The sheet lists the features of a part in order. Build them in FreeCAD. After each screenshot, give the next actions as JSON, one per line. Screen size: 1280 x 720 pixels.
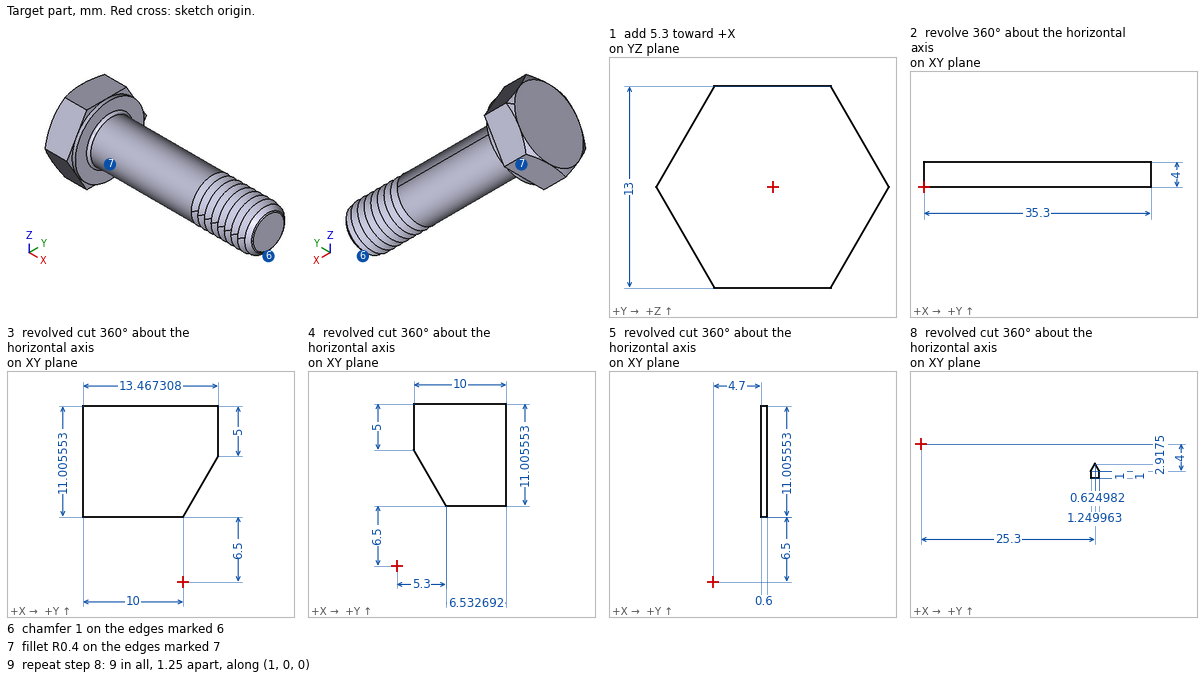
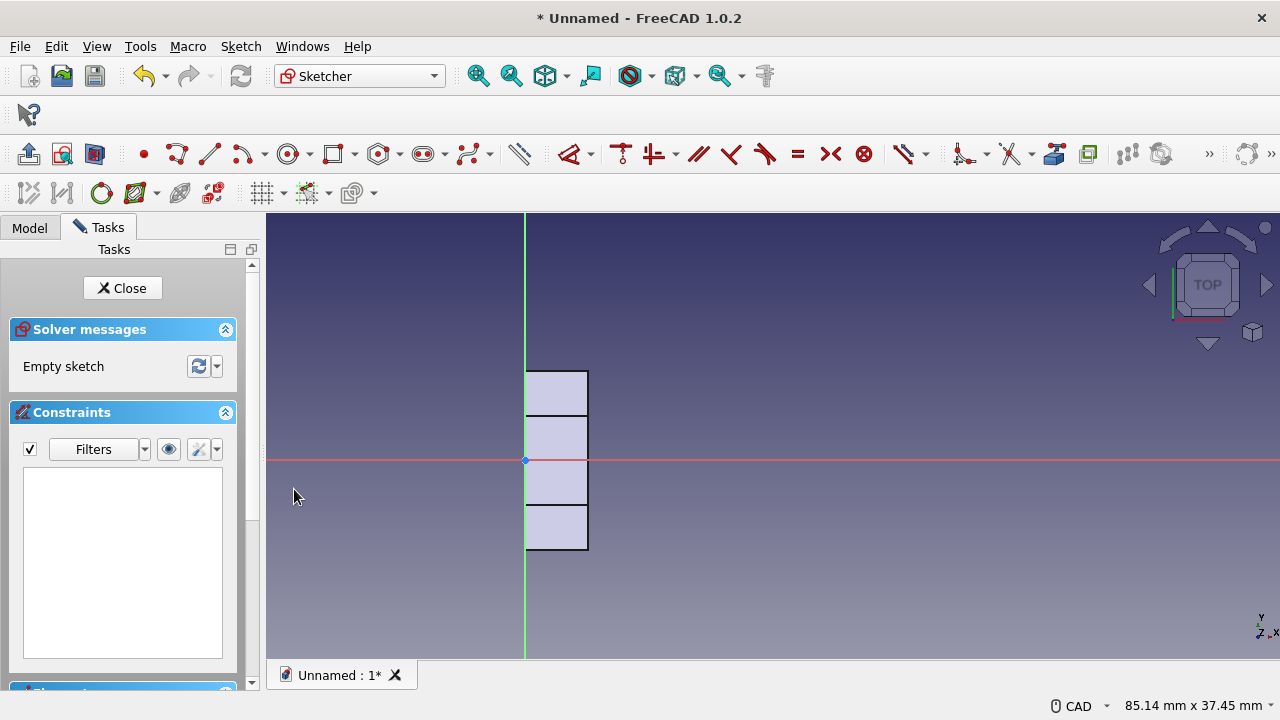
{"action": "scroll", "coordinate": [799, 437], "scroll_direction": "up", "scroll_amount": 2}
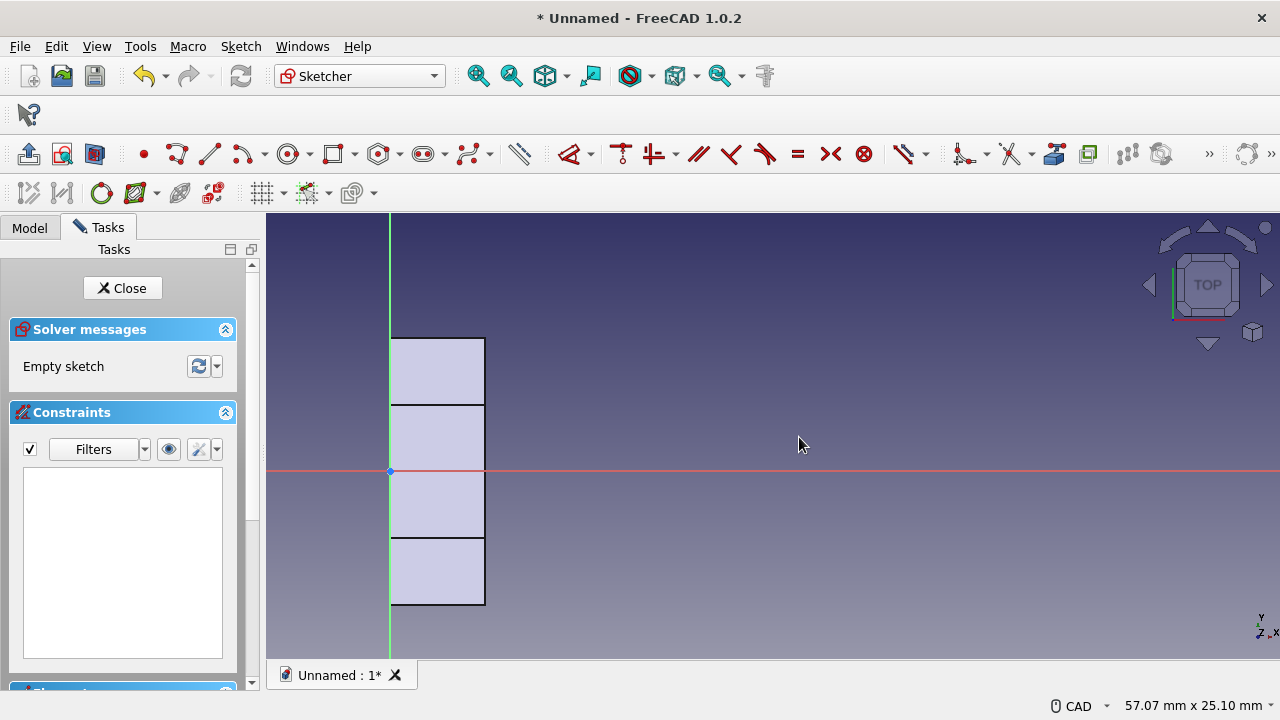
{"action": "left_click", "coordinate": [332, 154]}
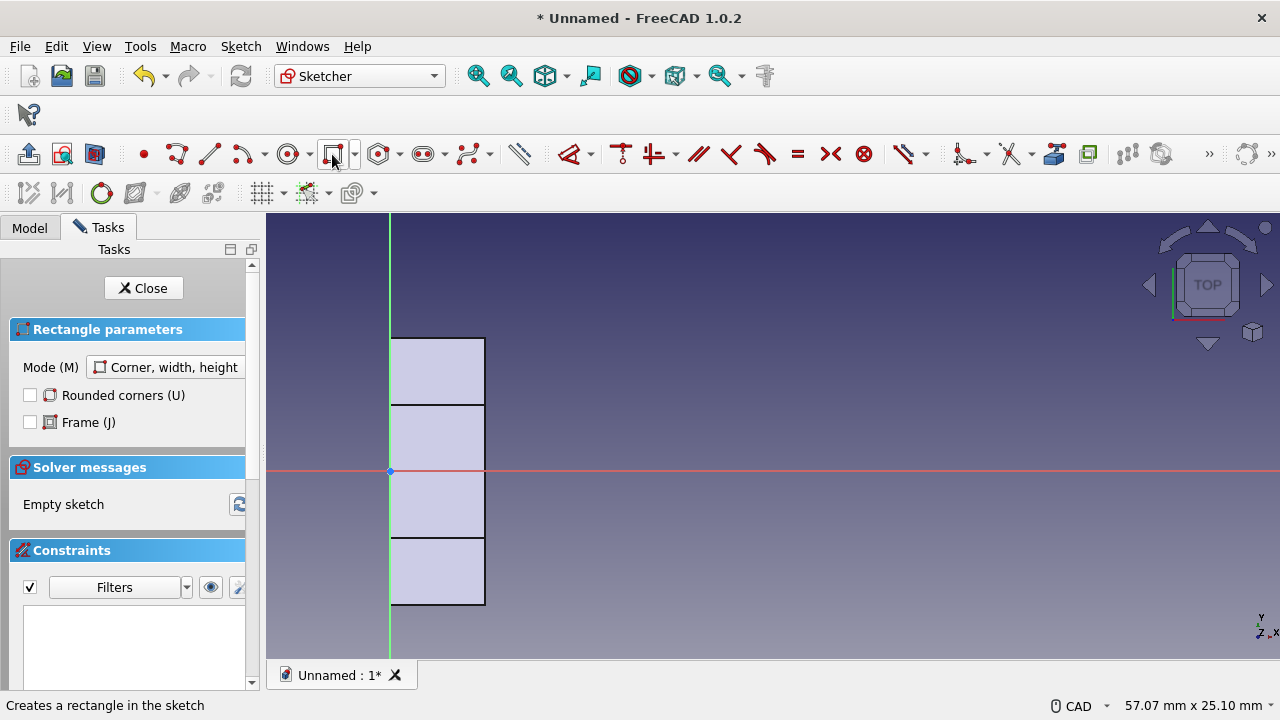
{"action": "left_click", "coordinate": [390, 471]}
{"action": "mouse_move", "coordinate": [1018, 400]}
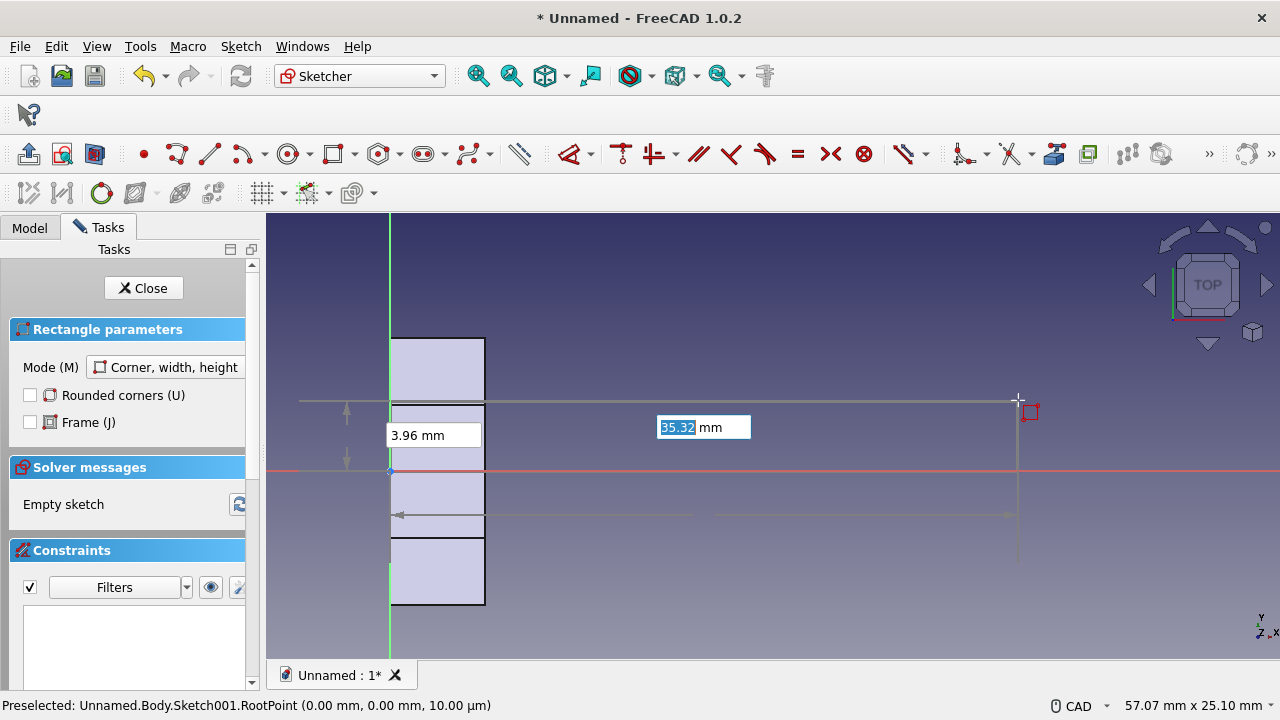
{"action": "type", "text": "35.3"}
{"action": "key", "text": "Tab"}
{"action": "type", "text": "4"}
{"action": "key", "text": "Return"}
{"action": "key", "text": "Escape"}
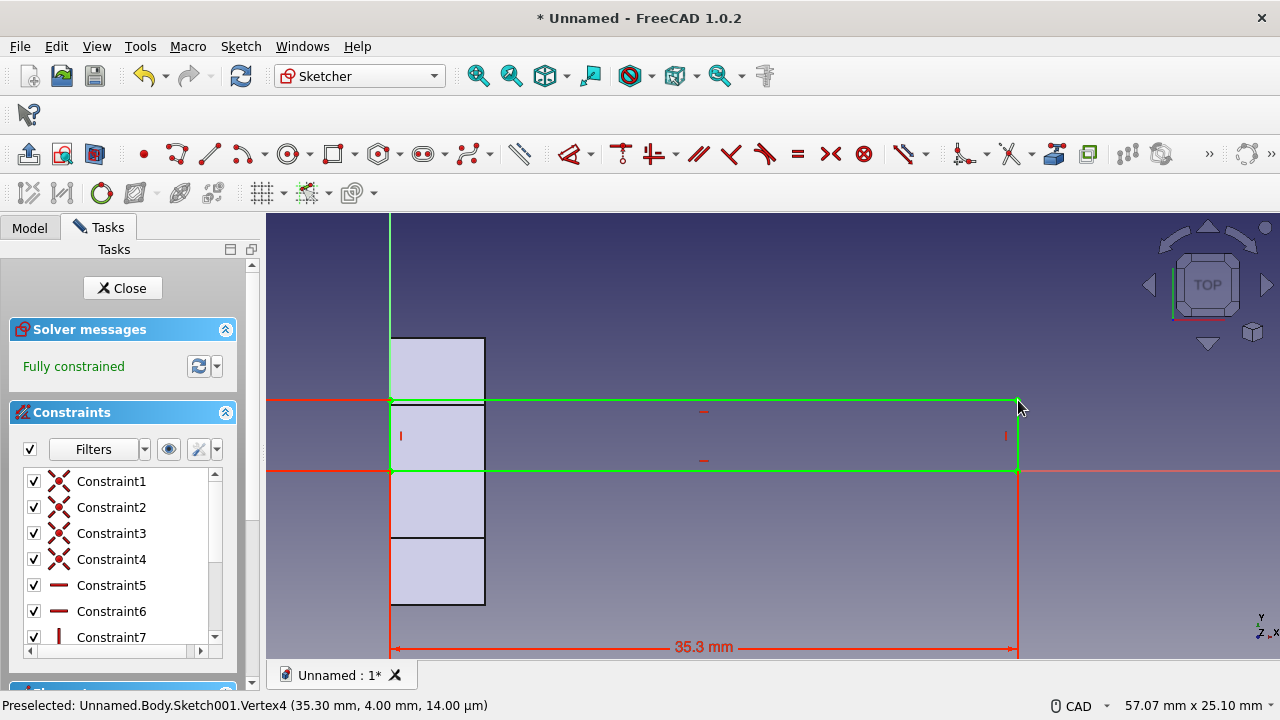
{"action": "left_click", "coordinate": [123, 288]}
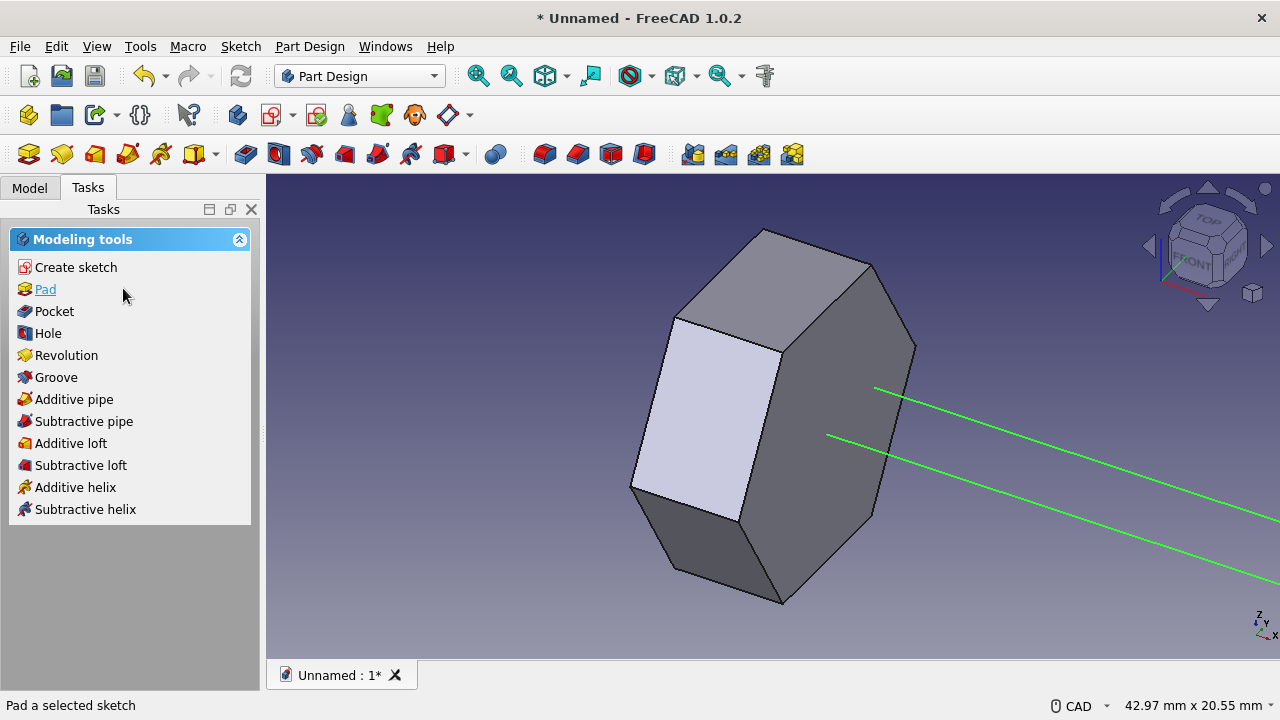
{"action": "left_click", "coordinate": [62, 154]}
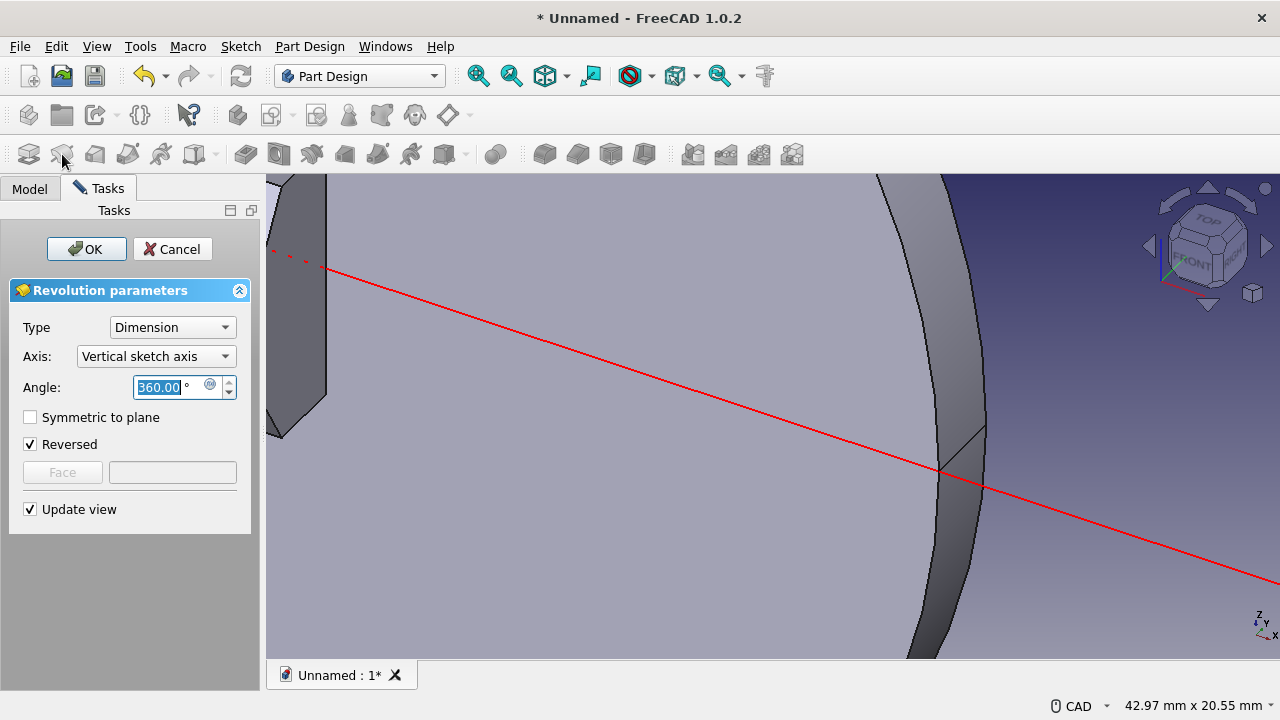
{"action": "left_click", "coordinate": [157, 356]}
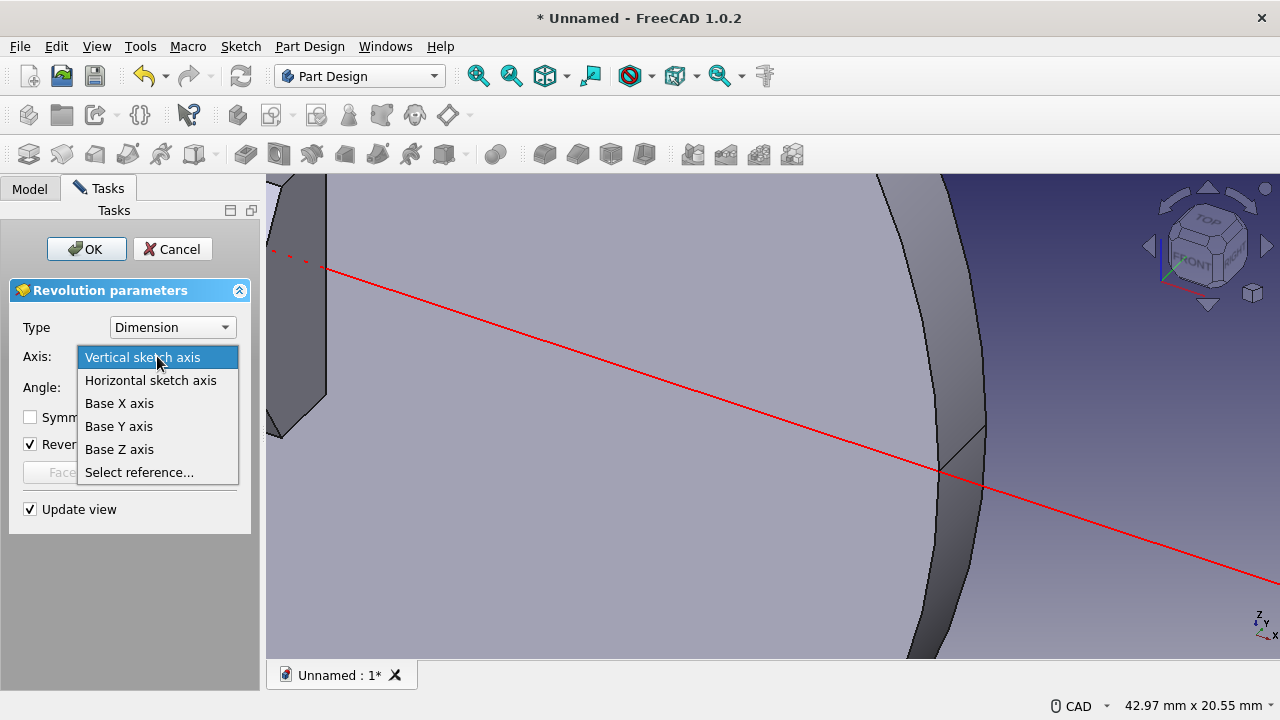
{"action": "left_click", "coordinate": [156, 380]}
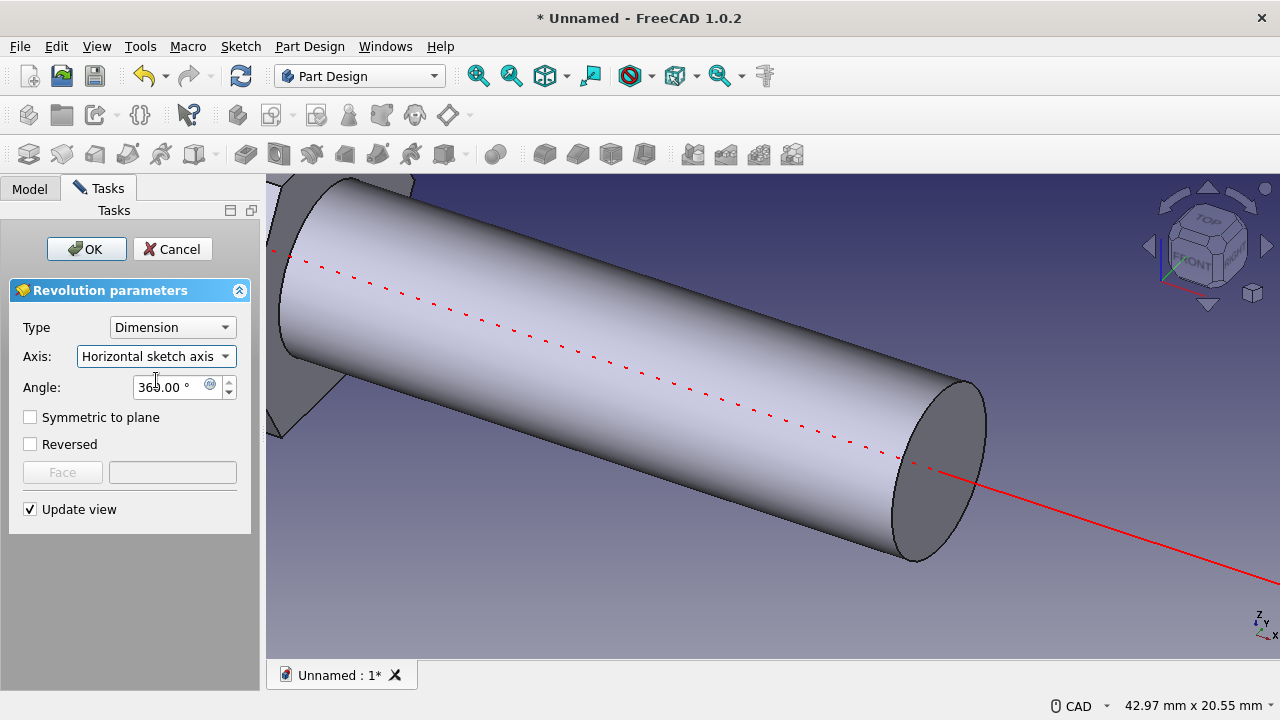
{"action": "left_click", "coordinate": [87, 249]}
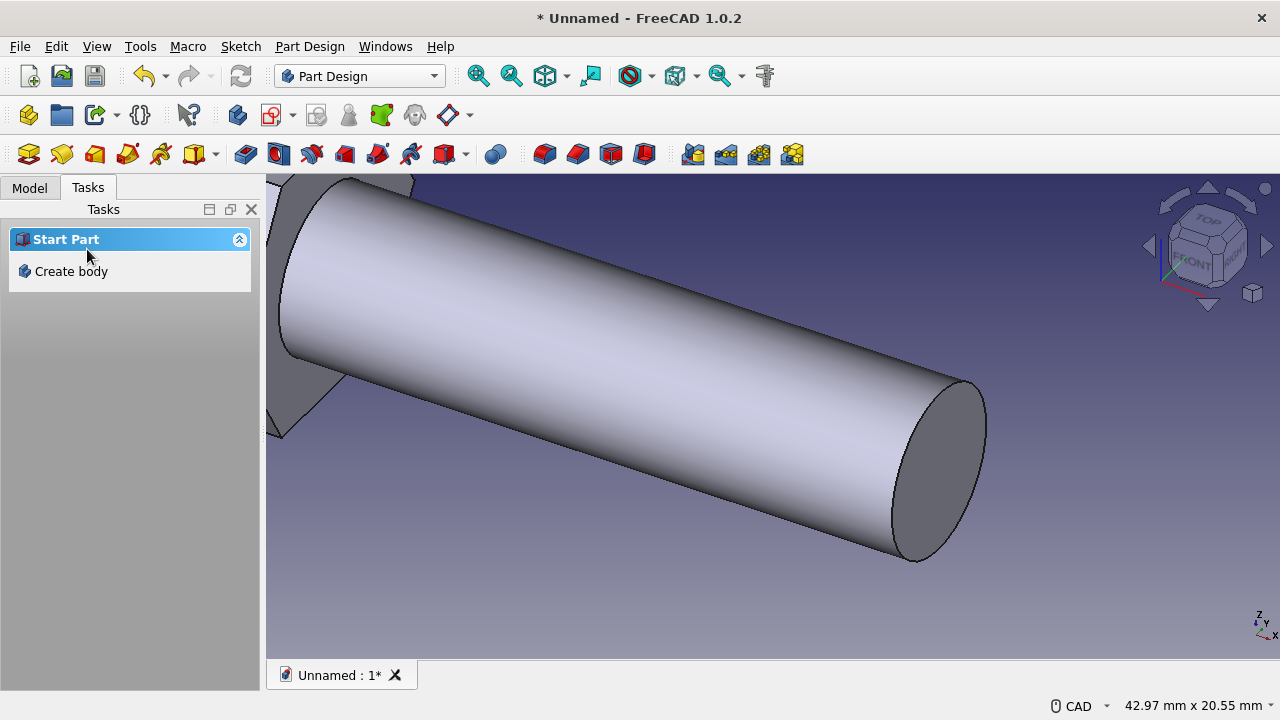
{"action": "key", "text": "v f"}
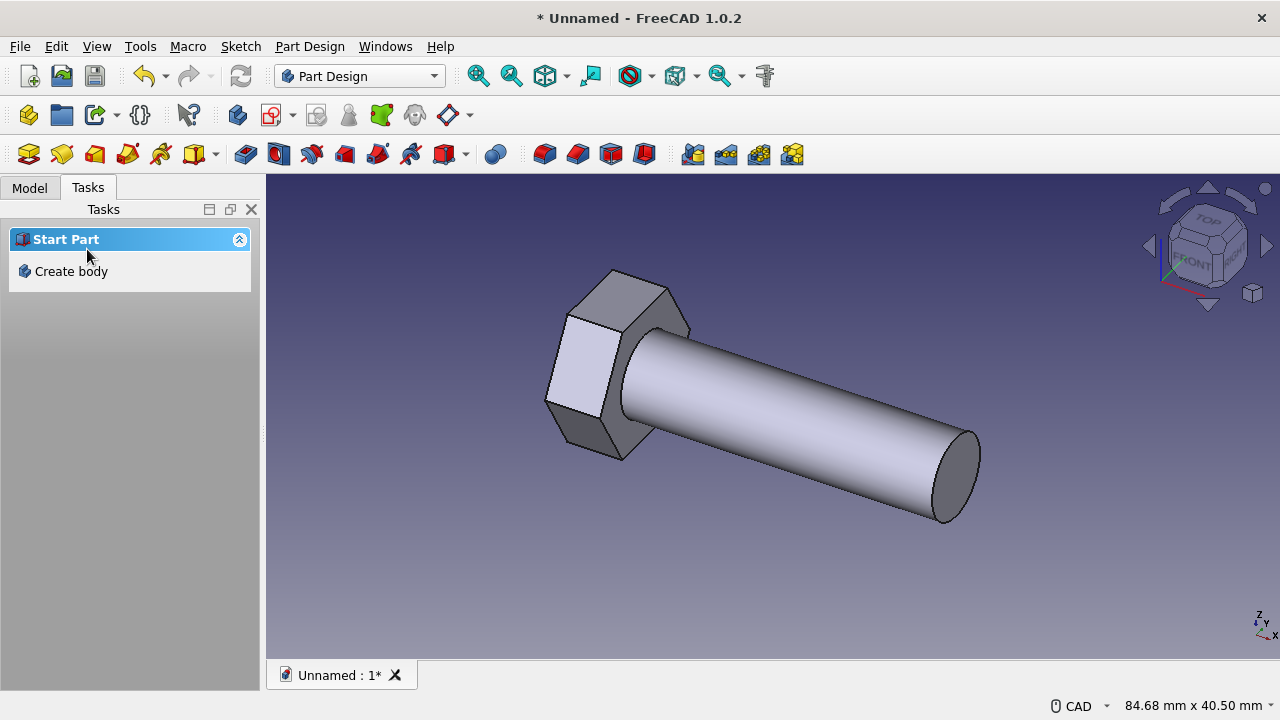
{"action": "left_click", "coordinate": [270, 116]}